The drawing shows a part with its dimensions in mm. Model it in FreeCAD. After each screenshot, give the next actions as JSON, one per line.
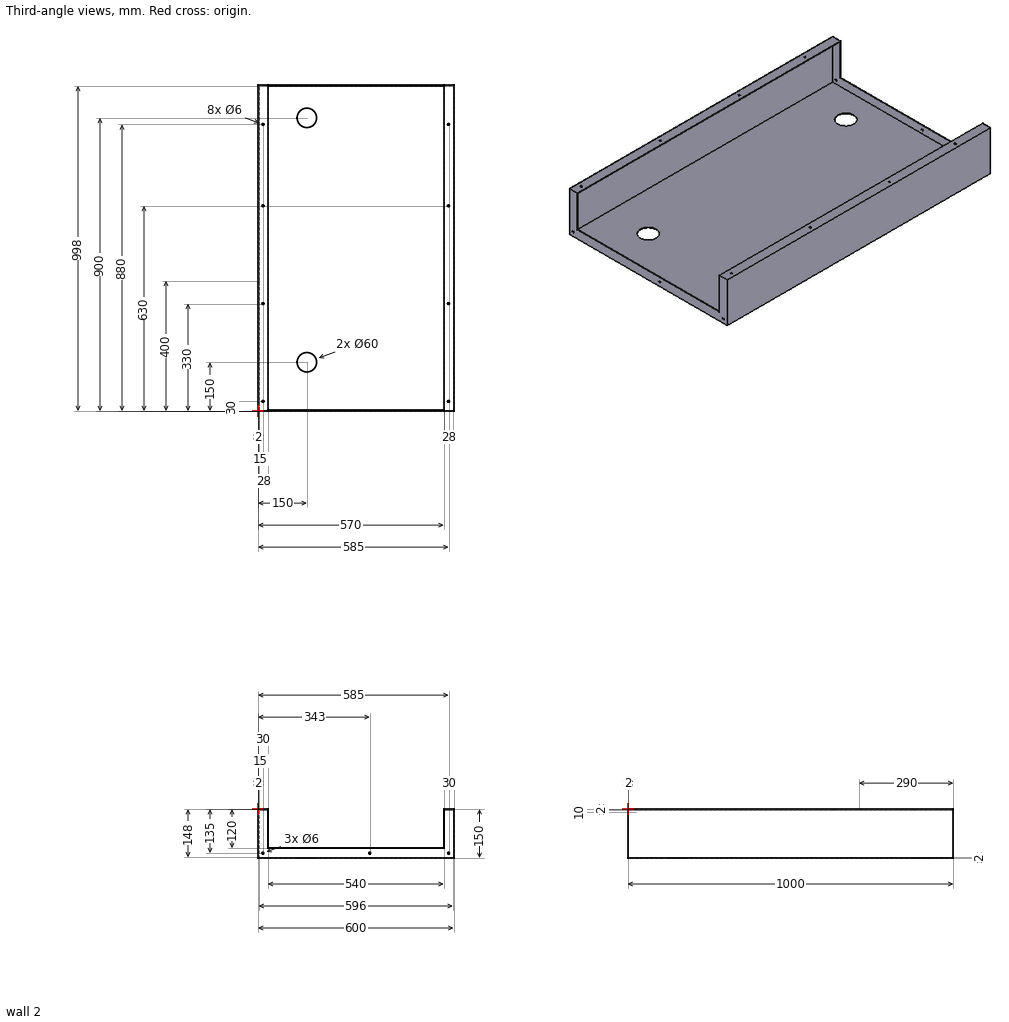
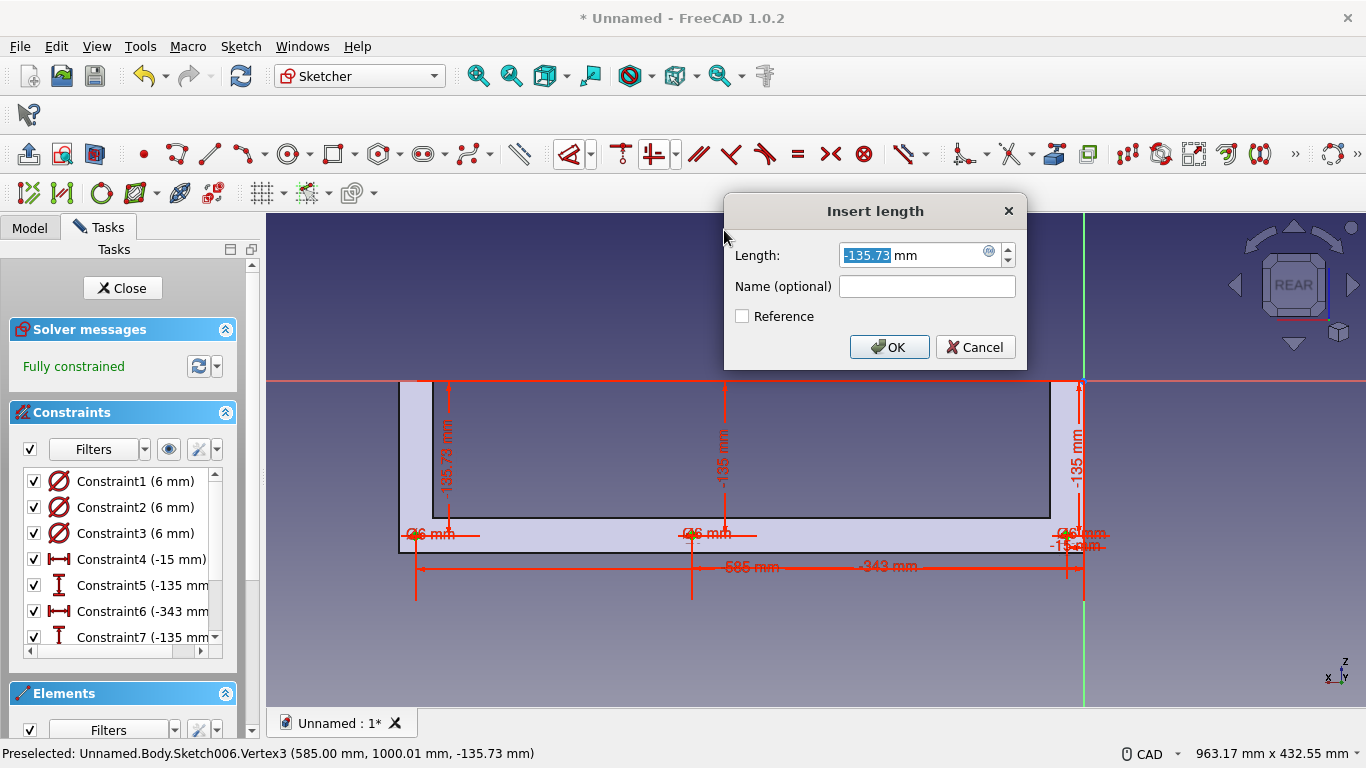
{"action": "type", "text": "-135"}
{"action": "key", "text": "Return"}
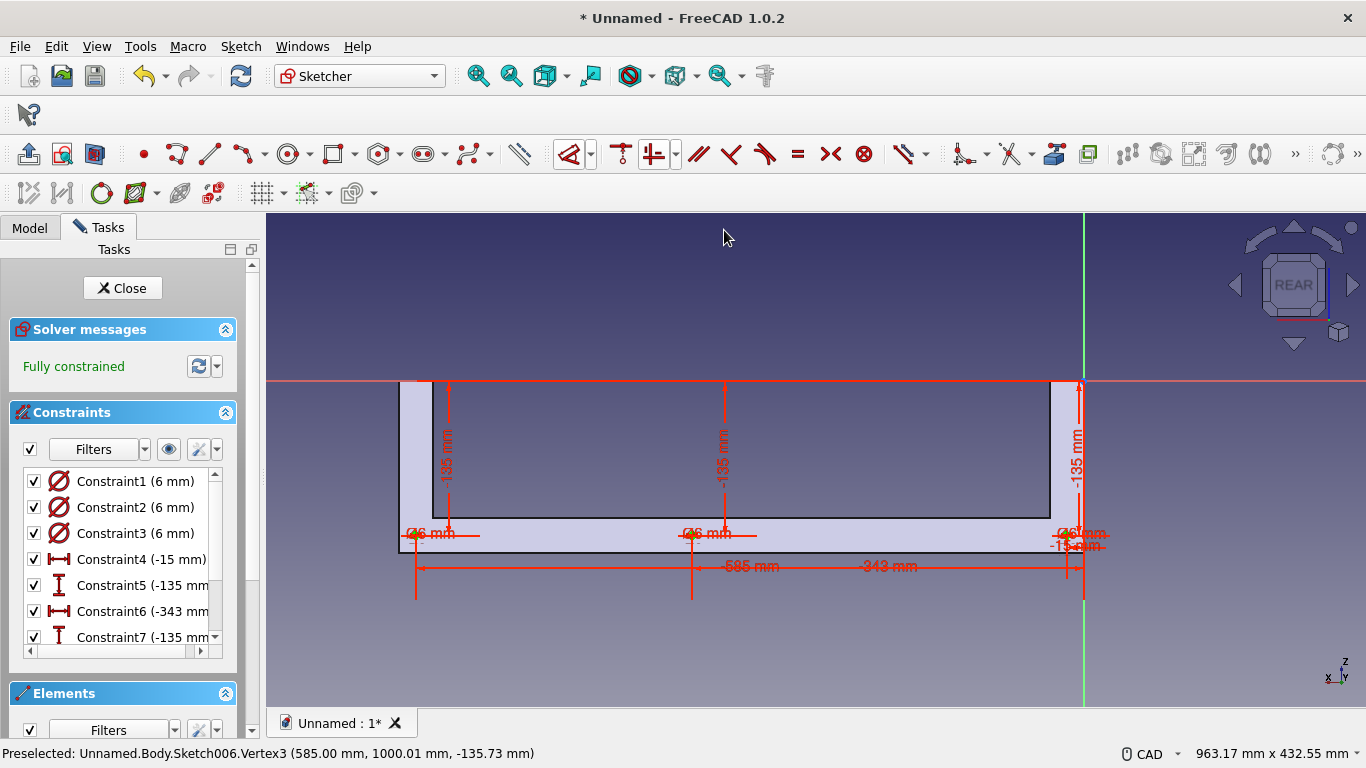
{"action": "left_click", "coordinate": [123, 288]}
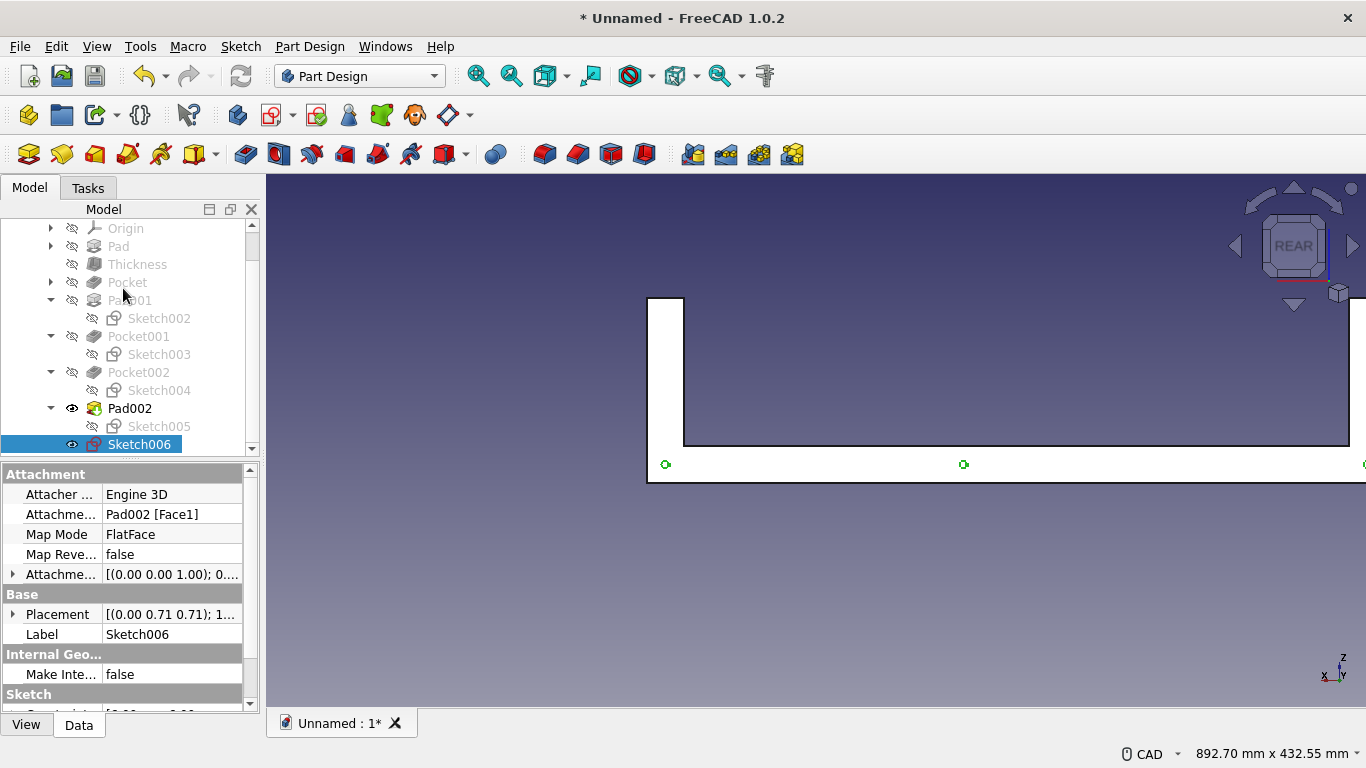
{"action": "left_click", "coordinate": [246, 154]}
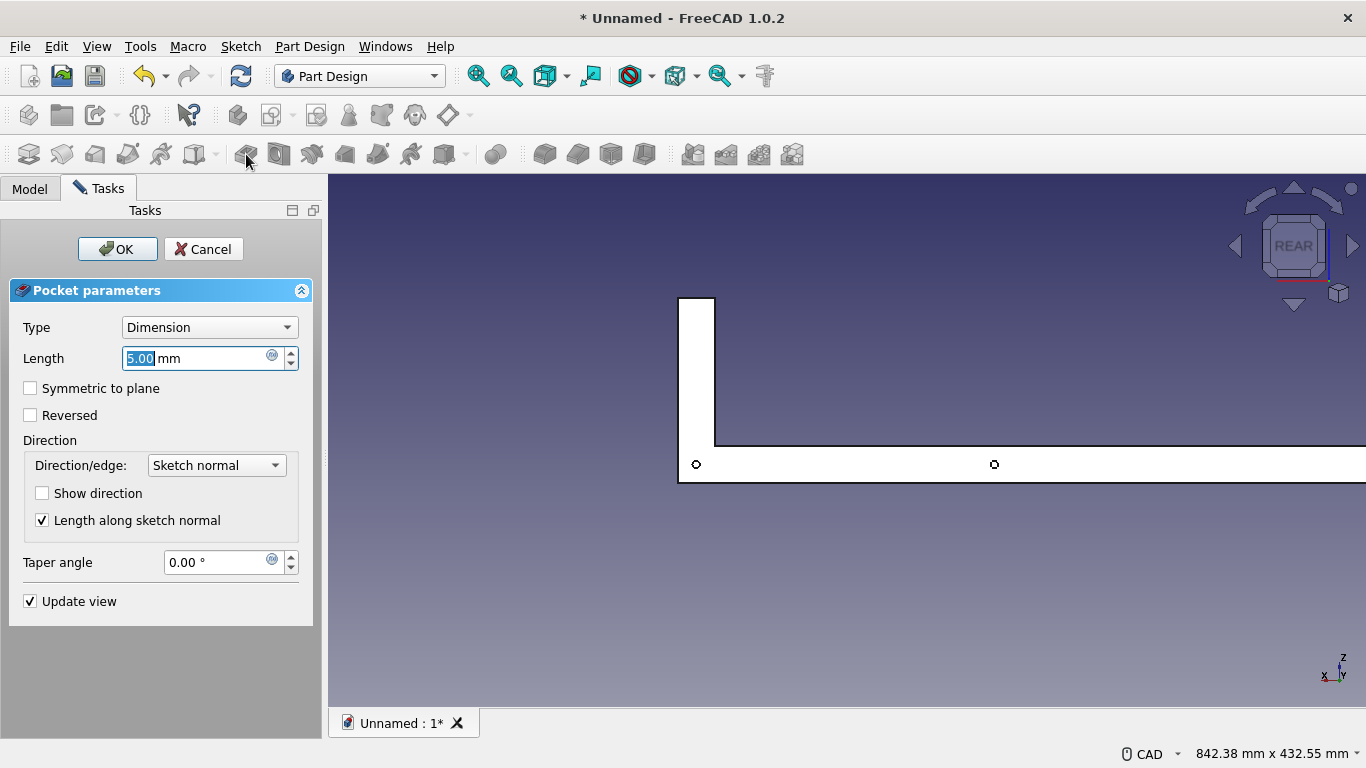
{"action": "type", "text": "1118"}
{"action": "key", "text": "Tab"}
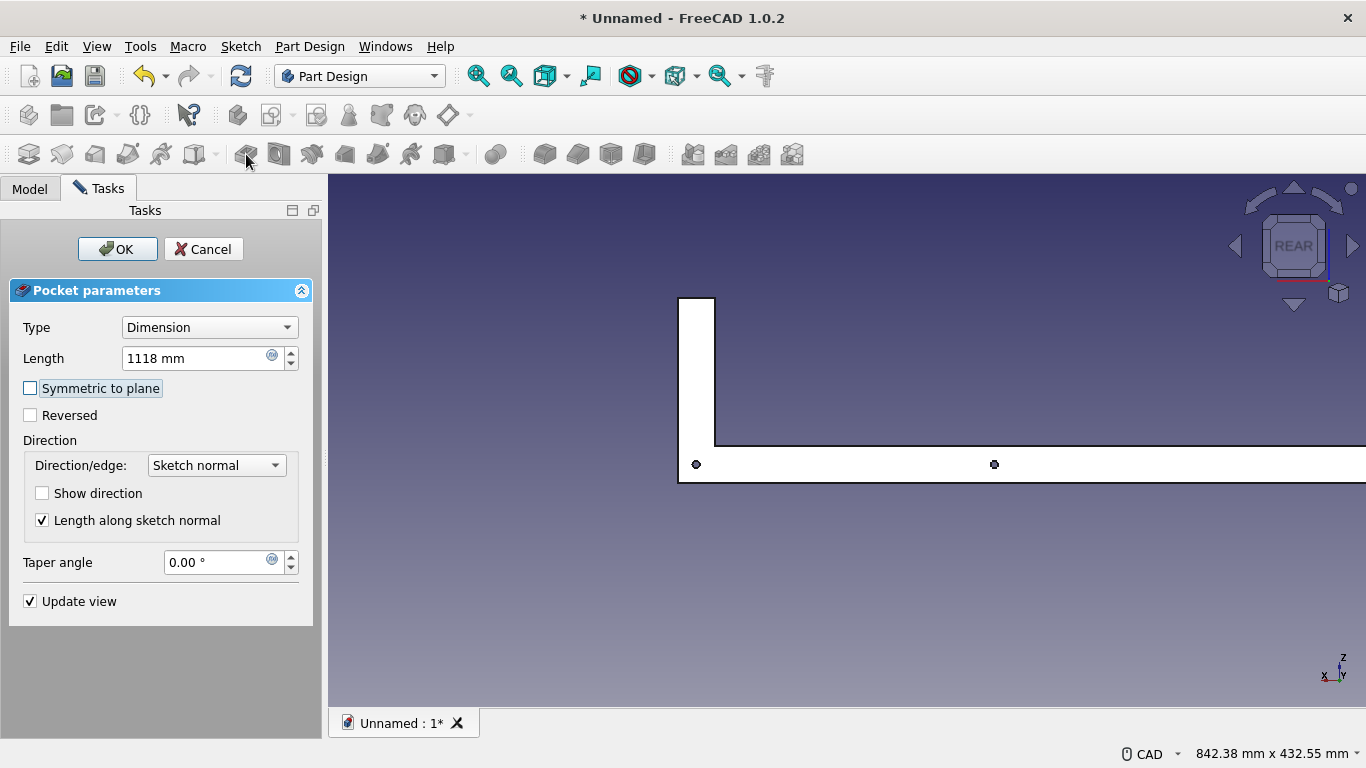
{"action": "left_click", "coordinate": [118, 249]}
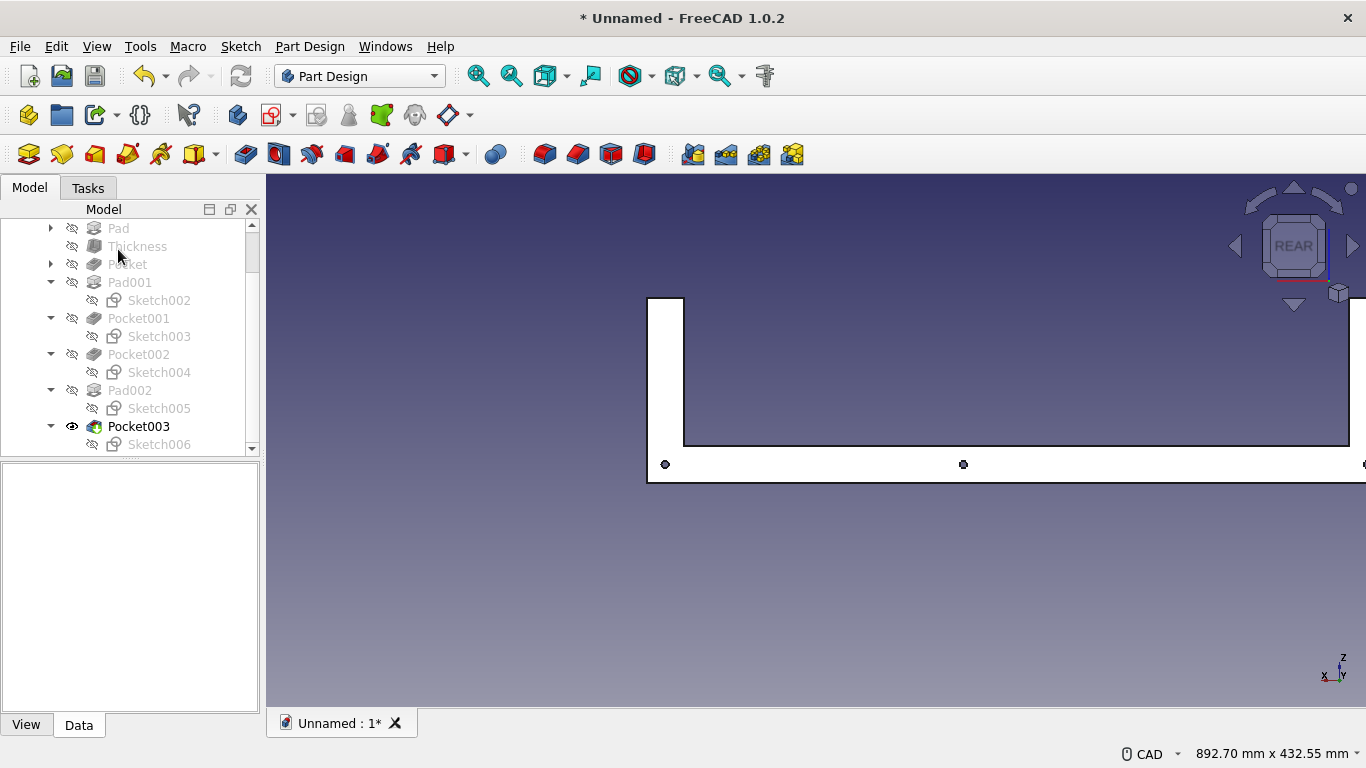
{"action": "left_click", "coordinate": [479, 76]}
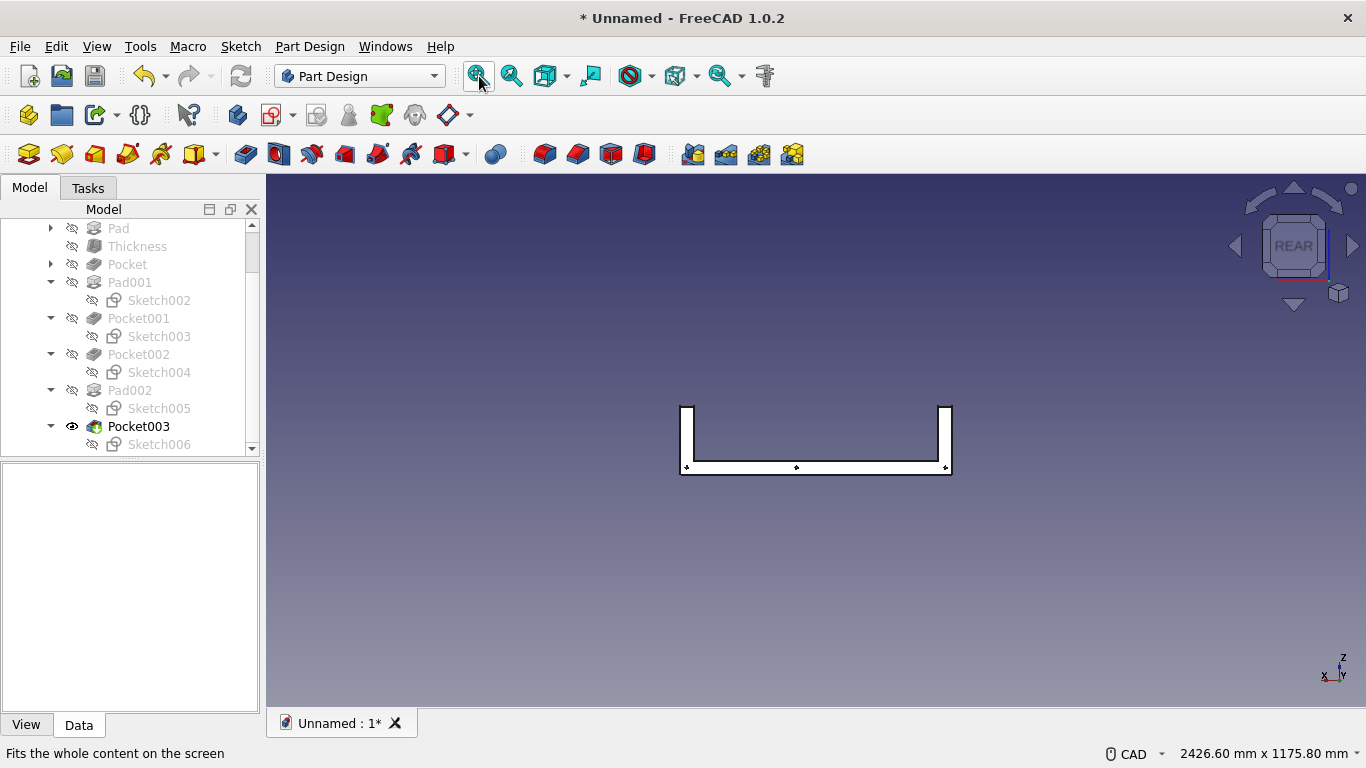
{"action": "left_click", "coordinate": [270, 116]}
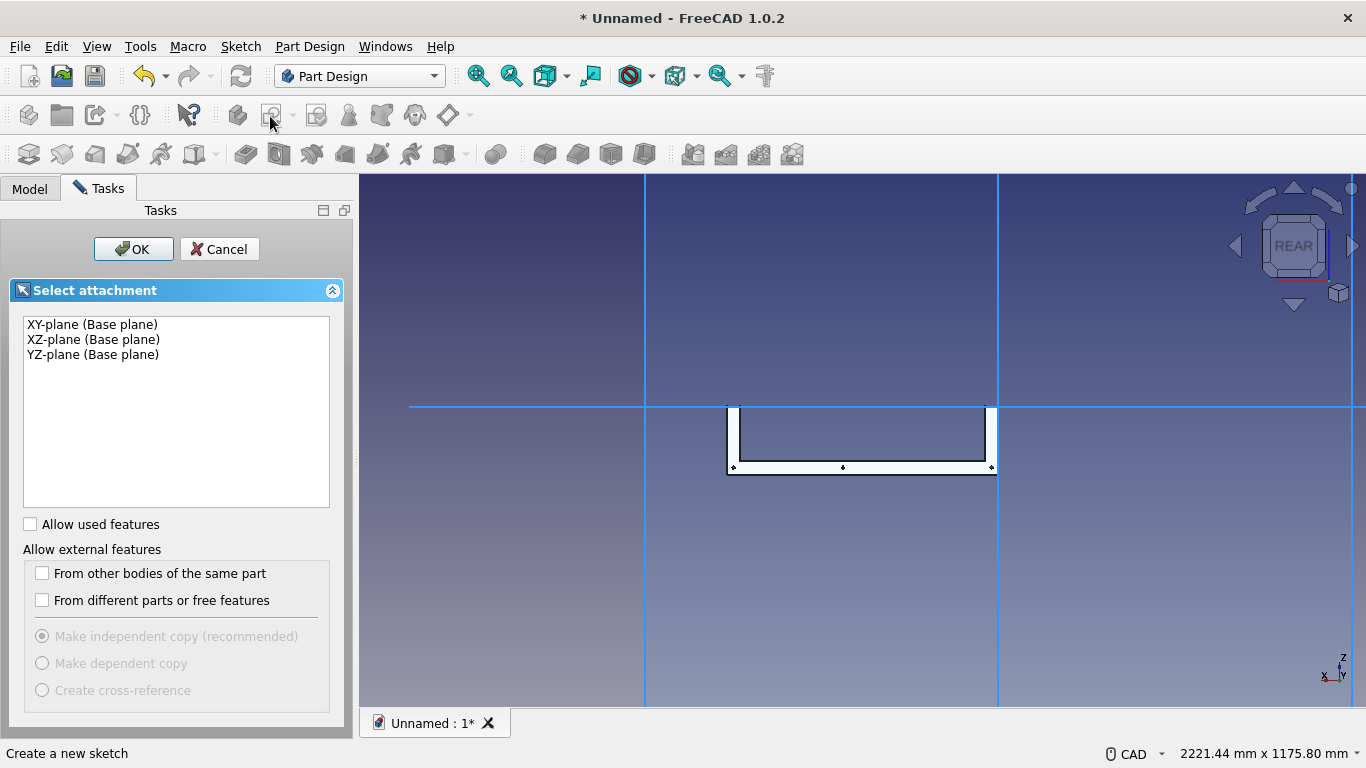
{"action": "left_click", "coordinate": [84, 324]}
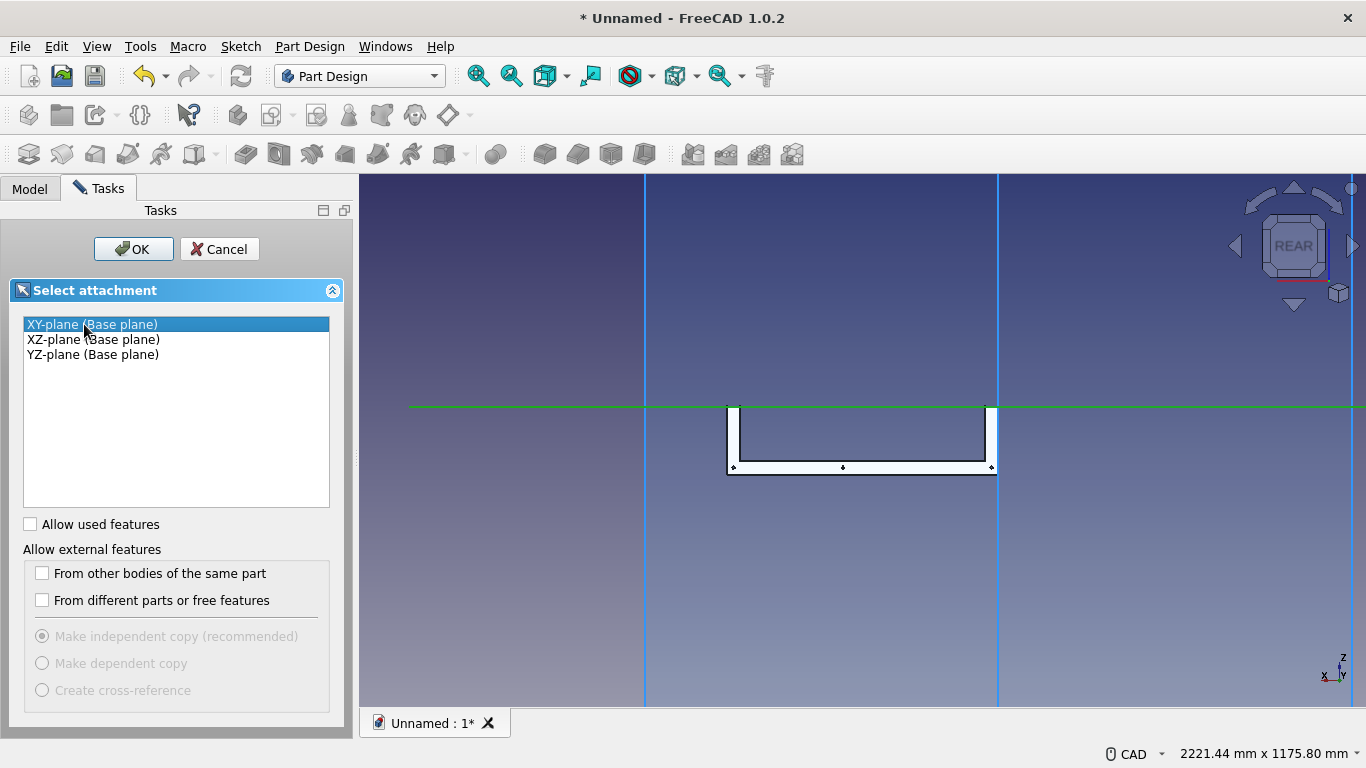
{"action": "left_click", "coordinate": [134, 249]}